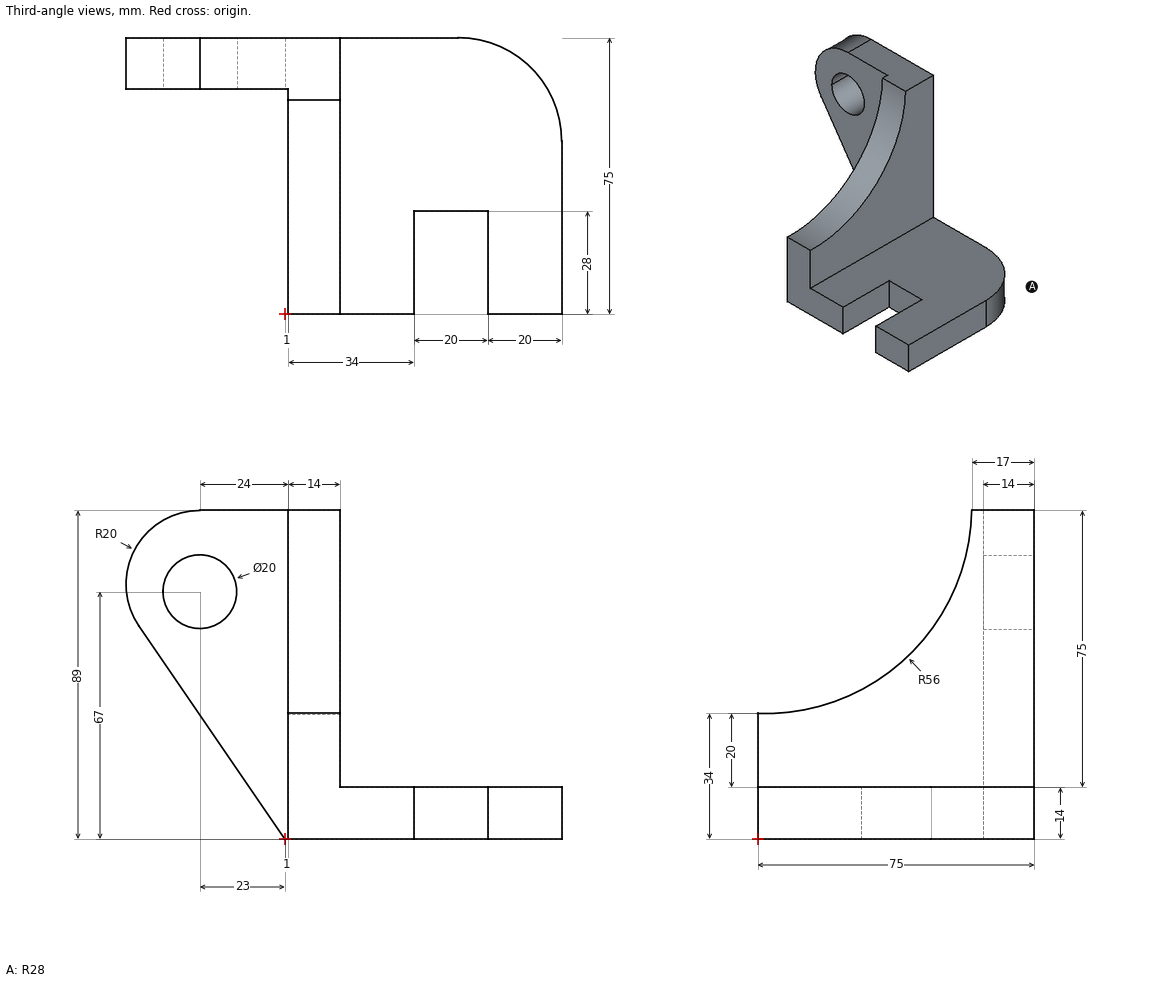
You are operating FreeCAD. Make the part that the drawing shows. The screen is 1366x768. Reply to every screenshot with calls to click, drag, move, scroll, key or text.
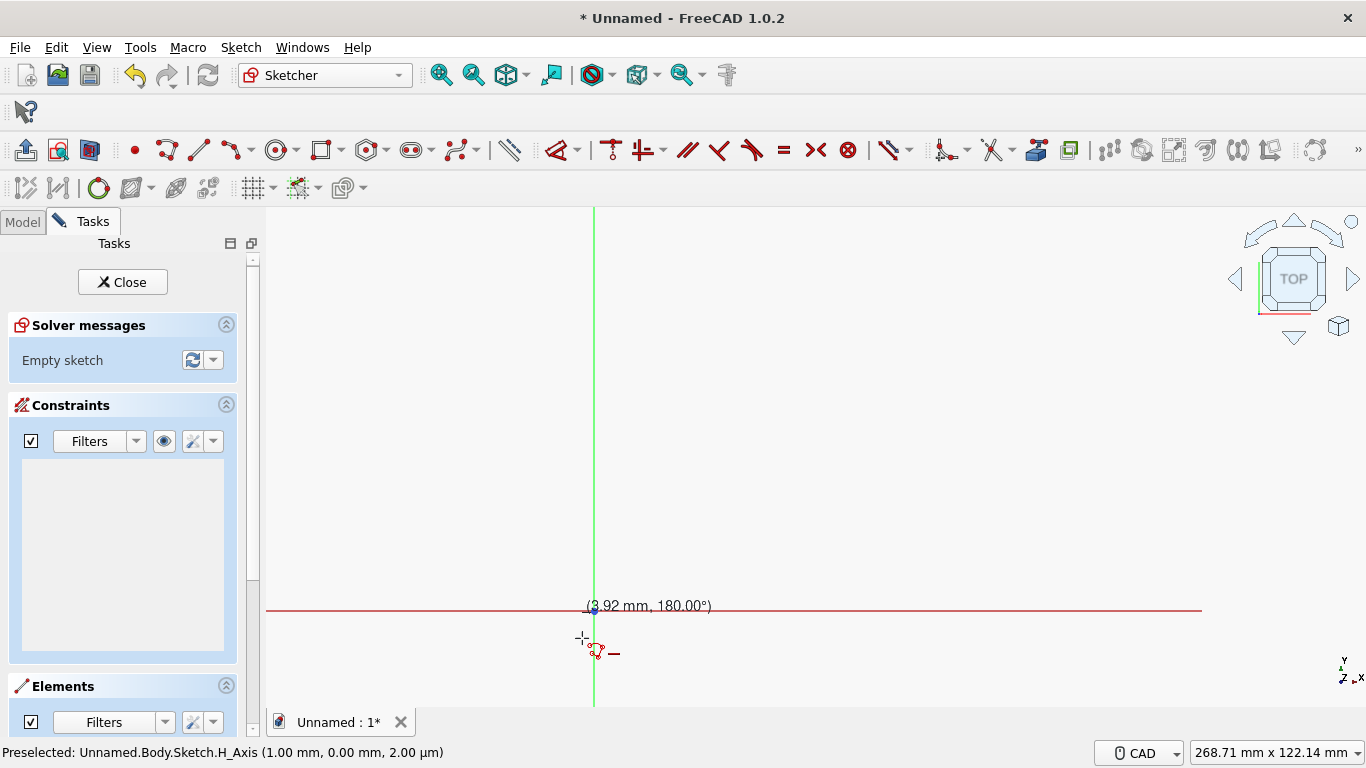
click(737, 602)
click(737, 496)
click(819, 496)
click(819, 611)
click(901, 602)
click(901, 304)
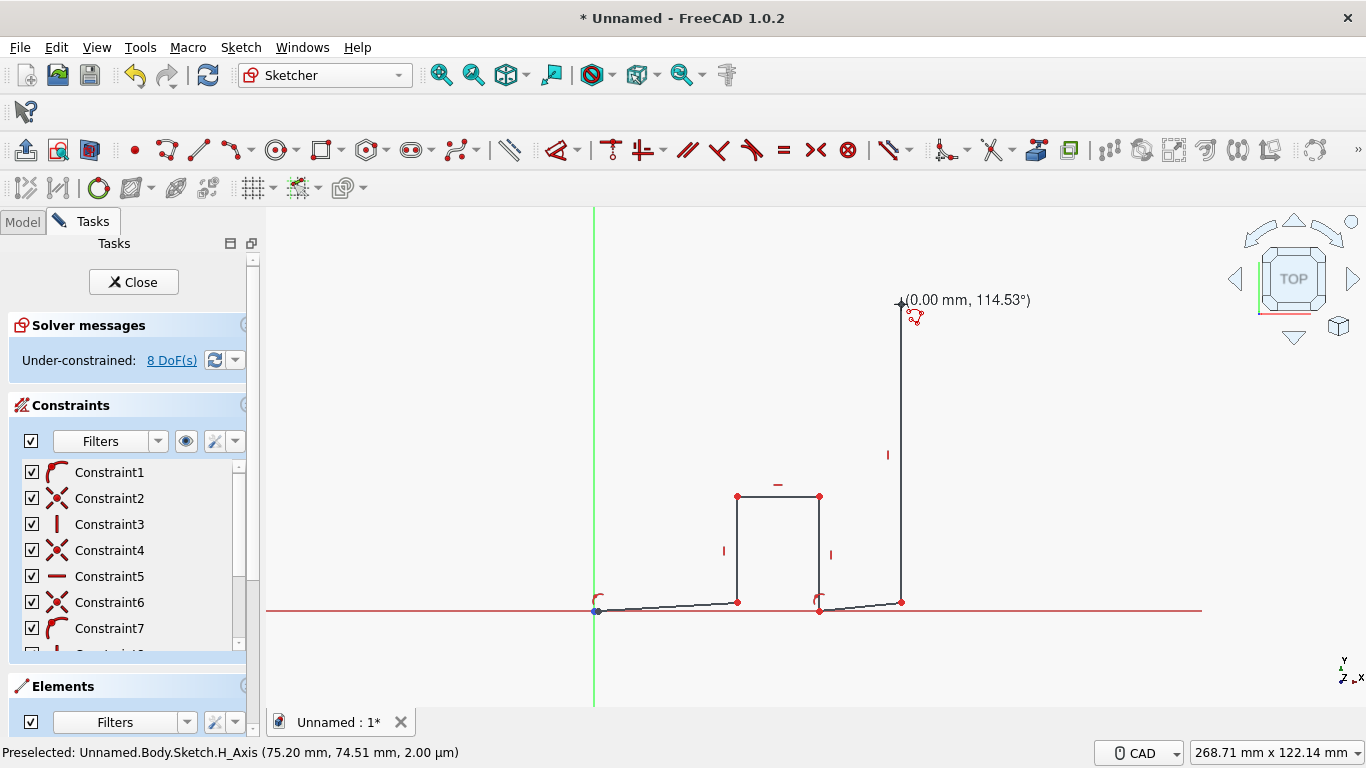
scroll(598, 304, up, 7)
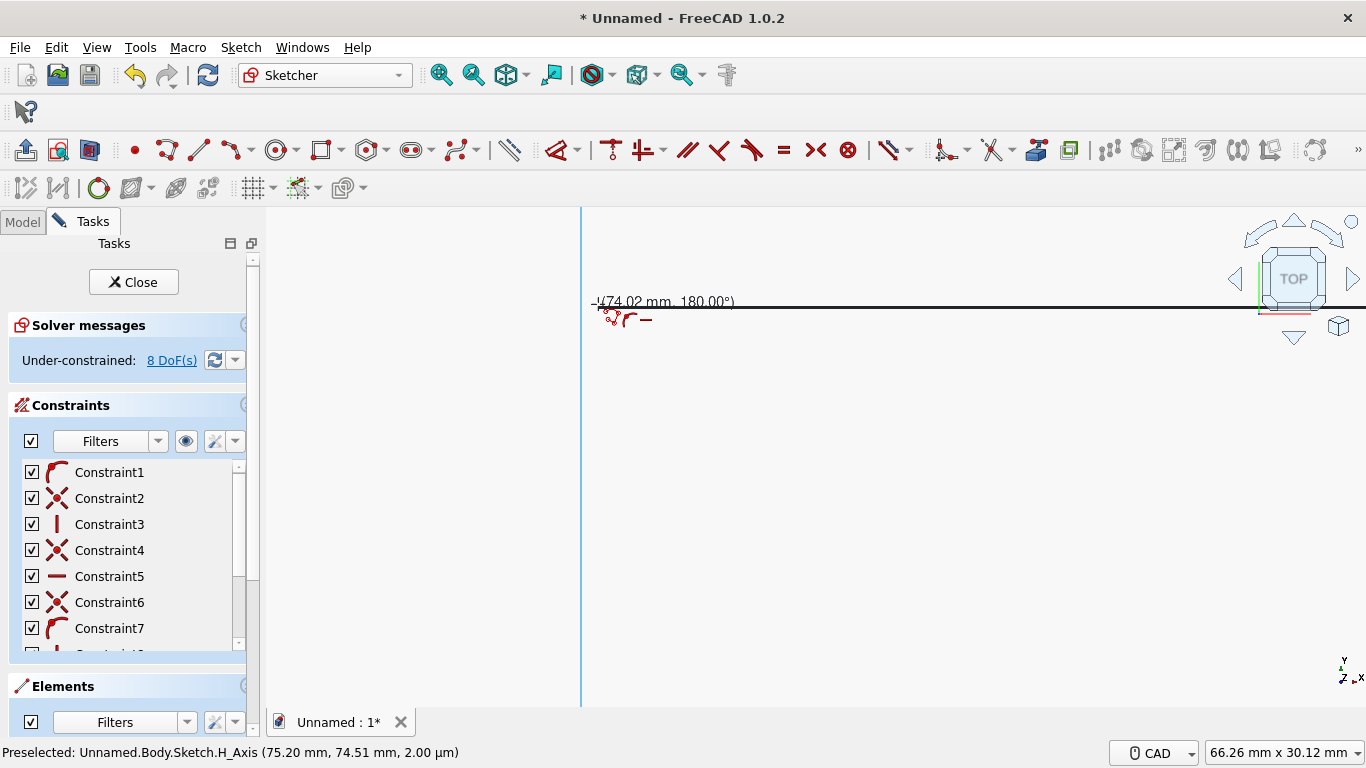
click(598, 303)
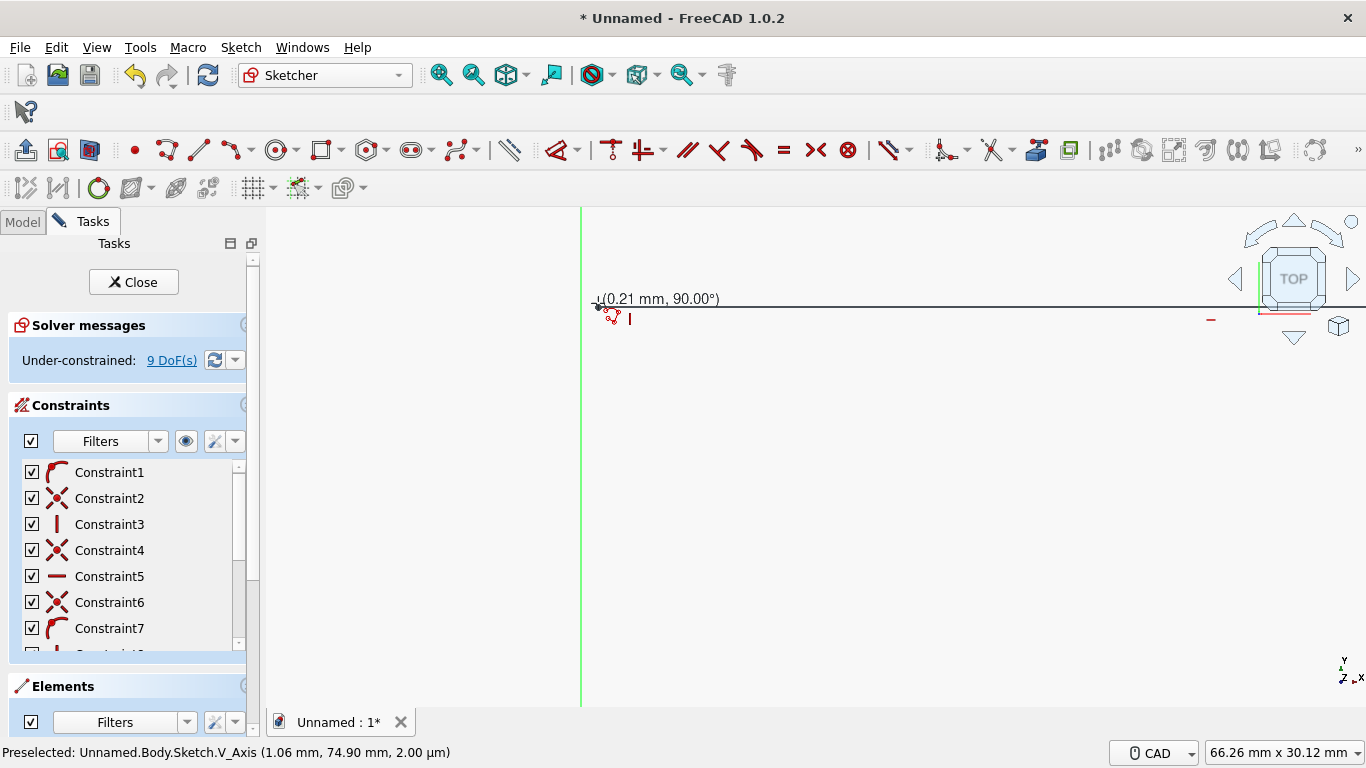
scroll(598, 304, down, 7)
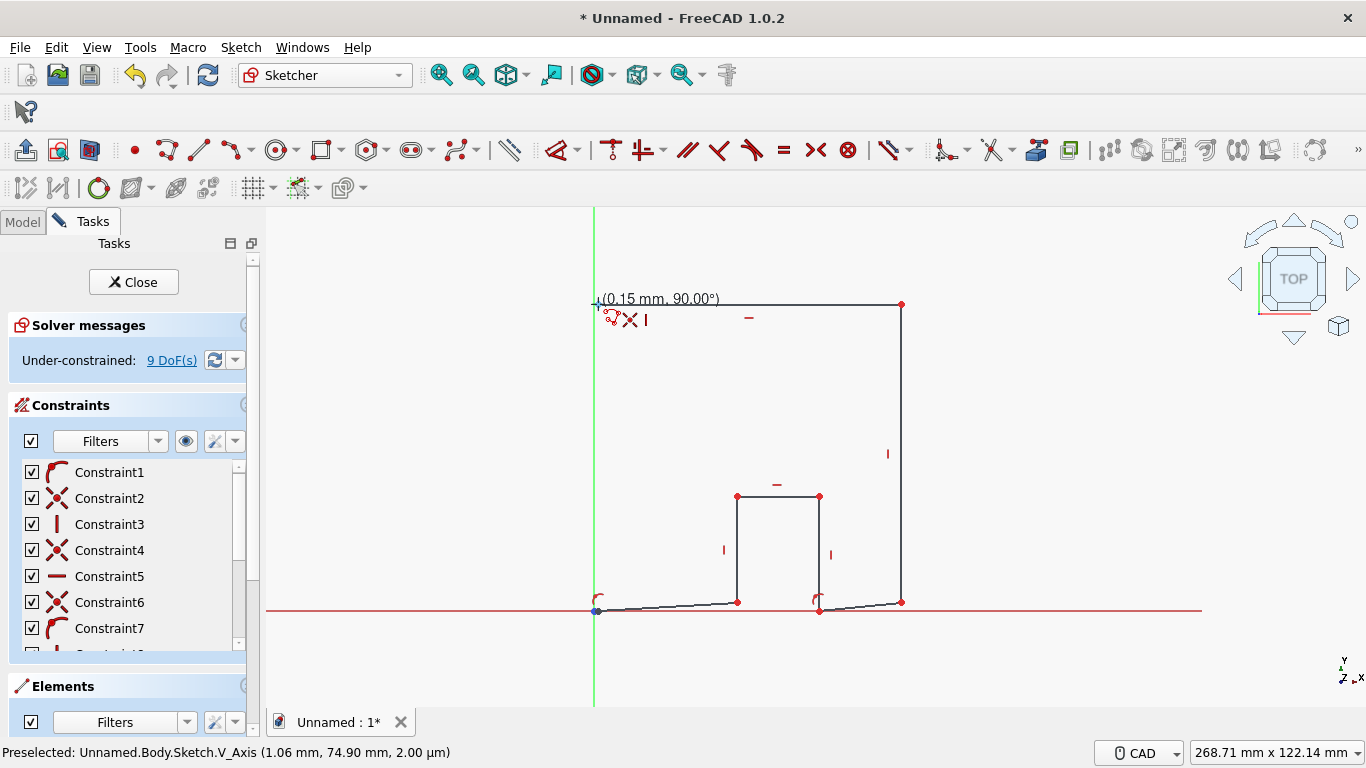
scroll(598, 611, up, 7)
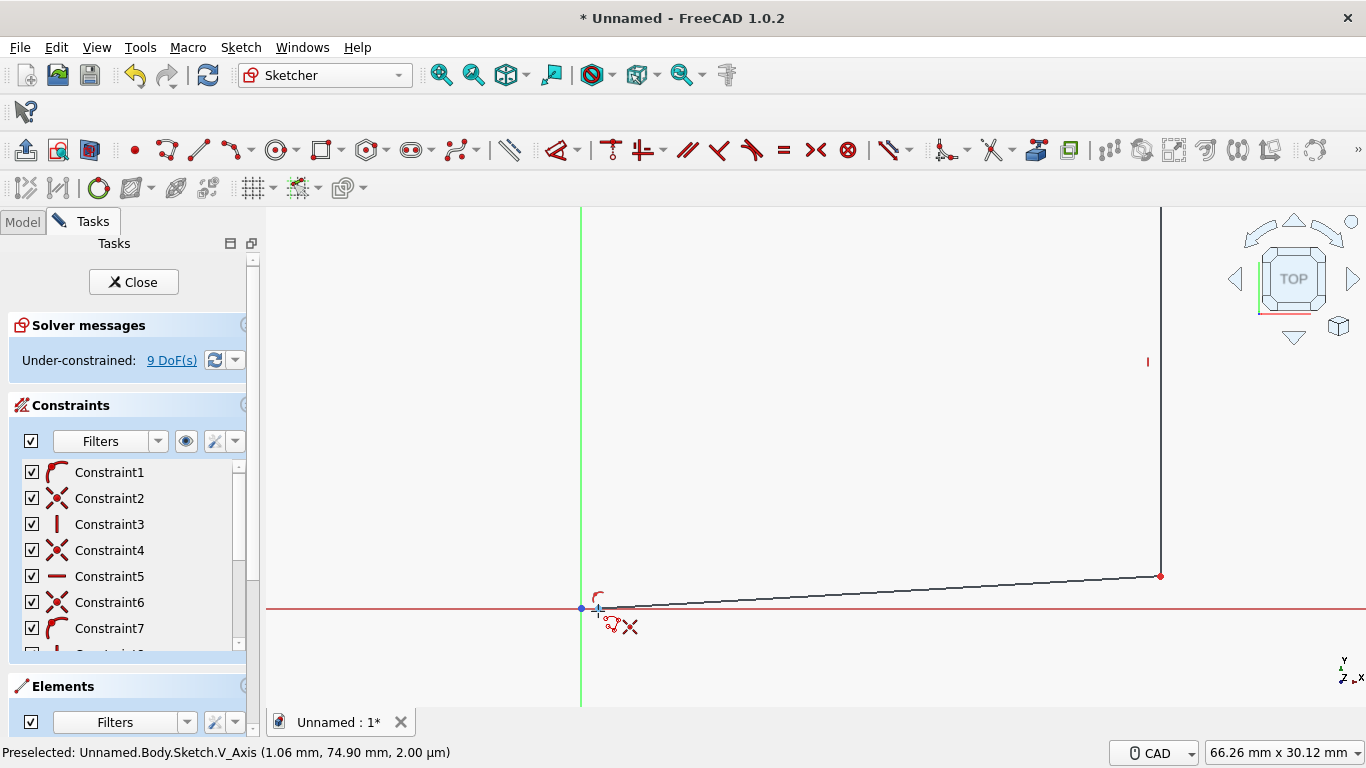
click(598, 609)
key(Escape)
key(Escape)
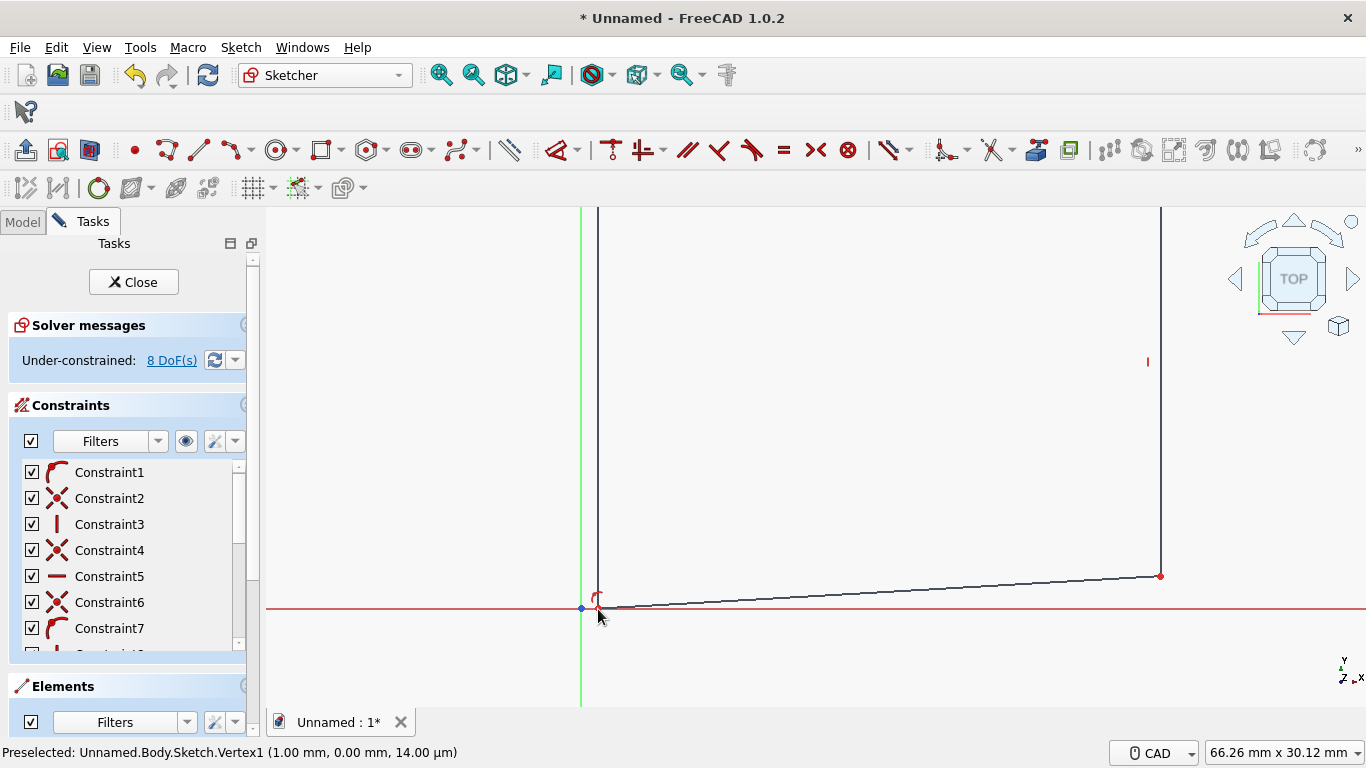
scroll(767, 599, up, 2)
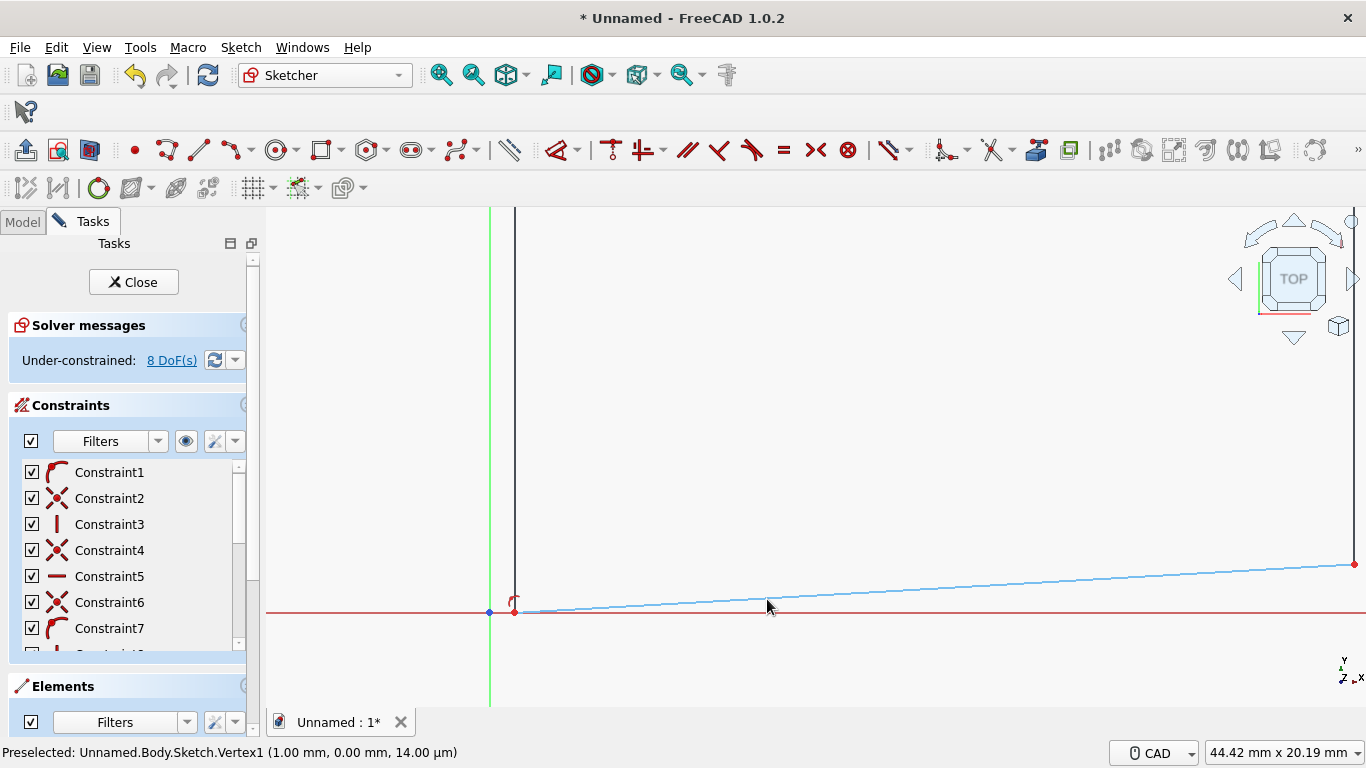
click(767, 598)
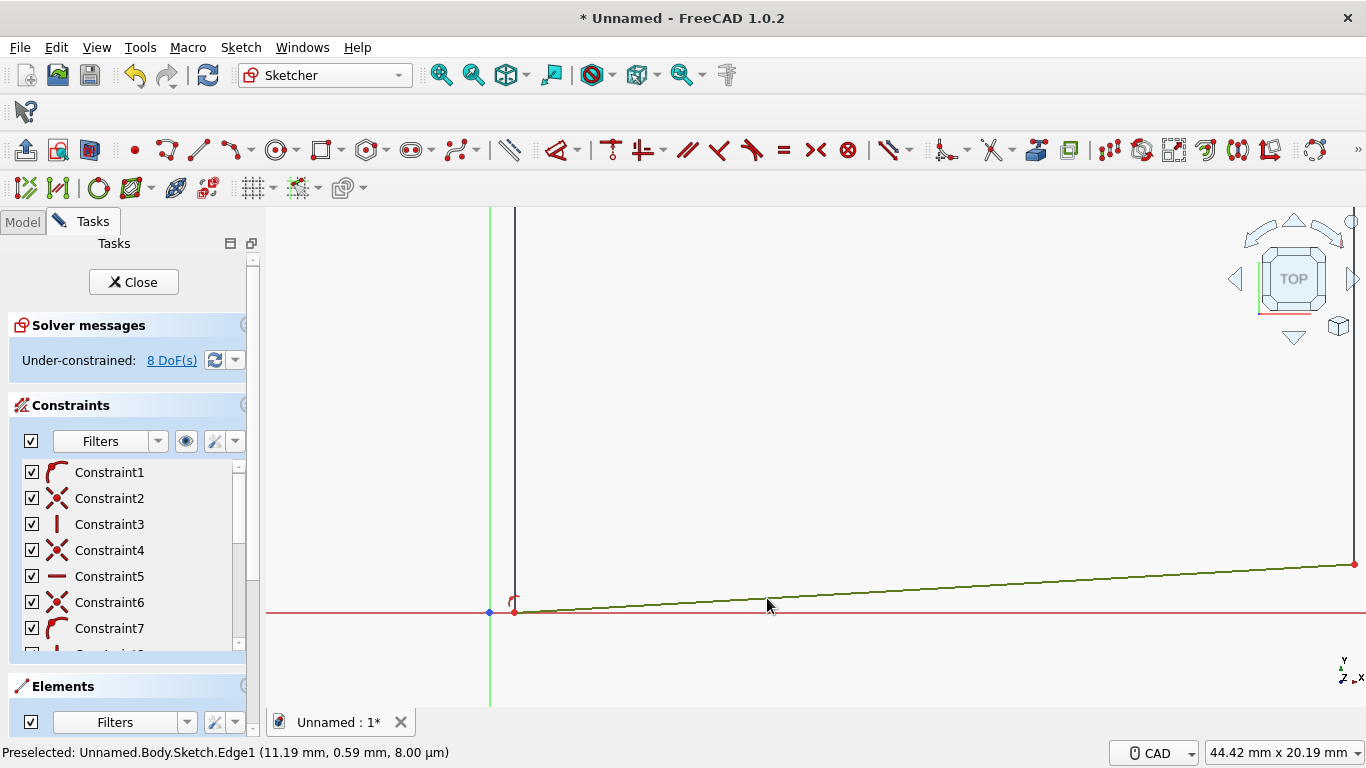
key(h)